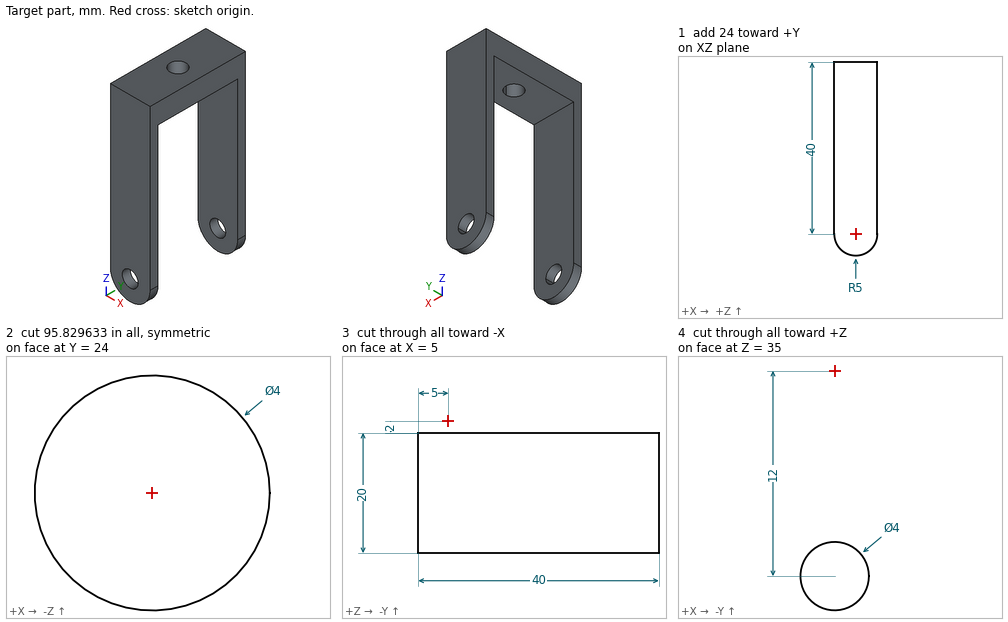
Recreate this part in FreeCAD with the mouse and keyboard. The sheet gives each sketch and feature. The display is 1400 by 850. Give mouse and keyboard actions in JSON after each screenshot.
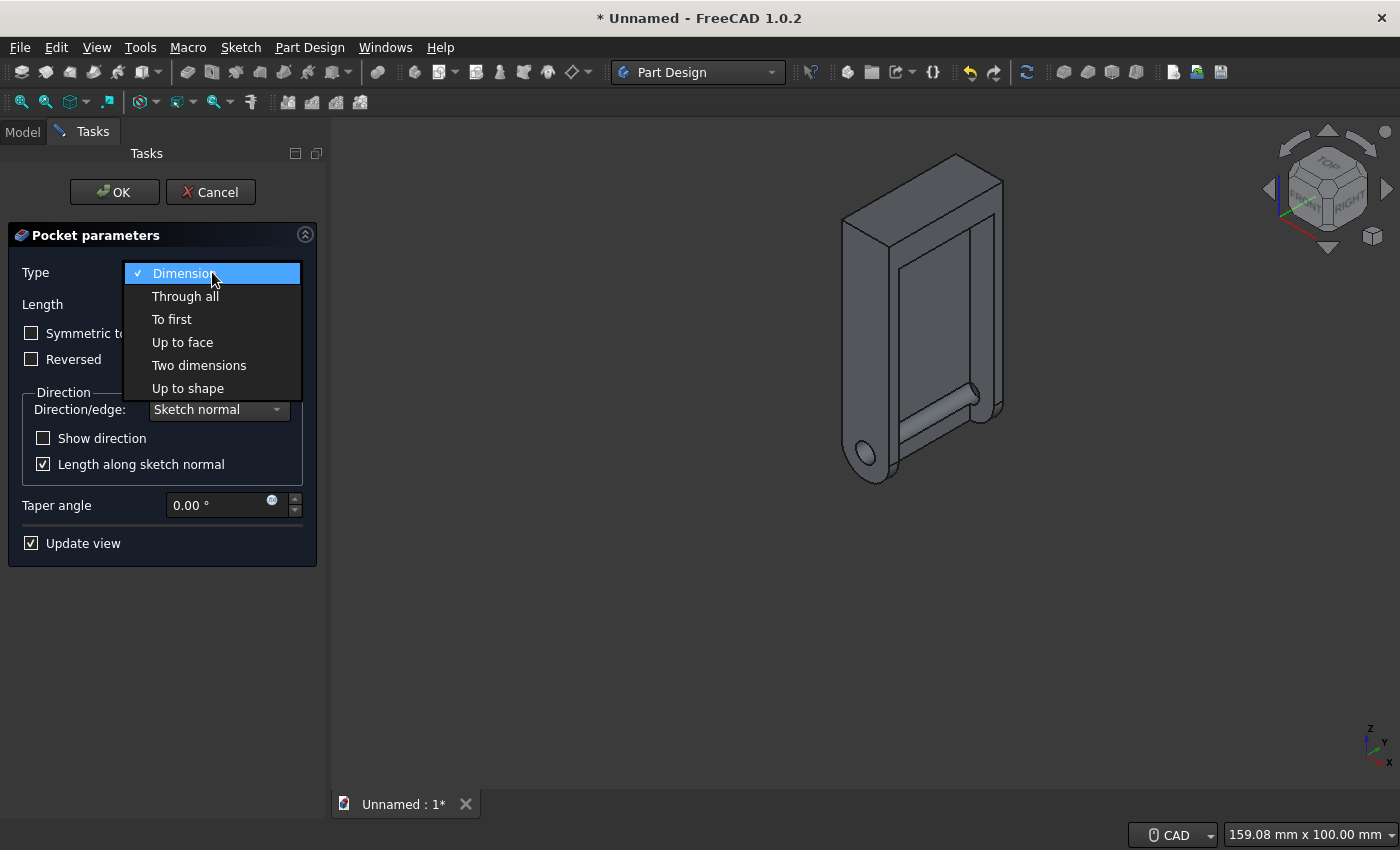
{"action": "left_click", "coordinate": [212, 296]}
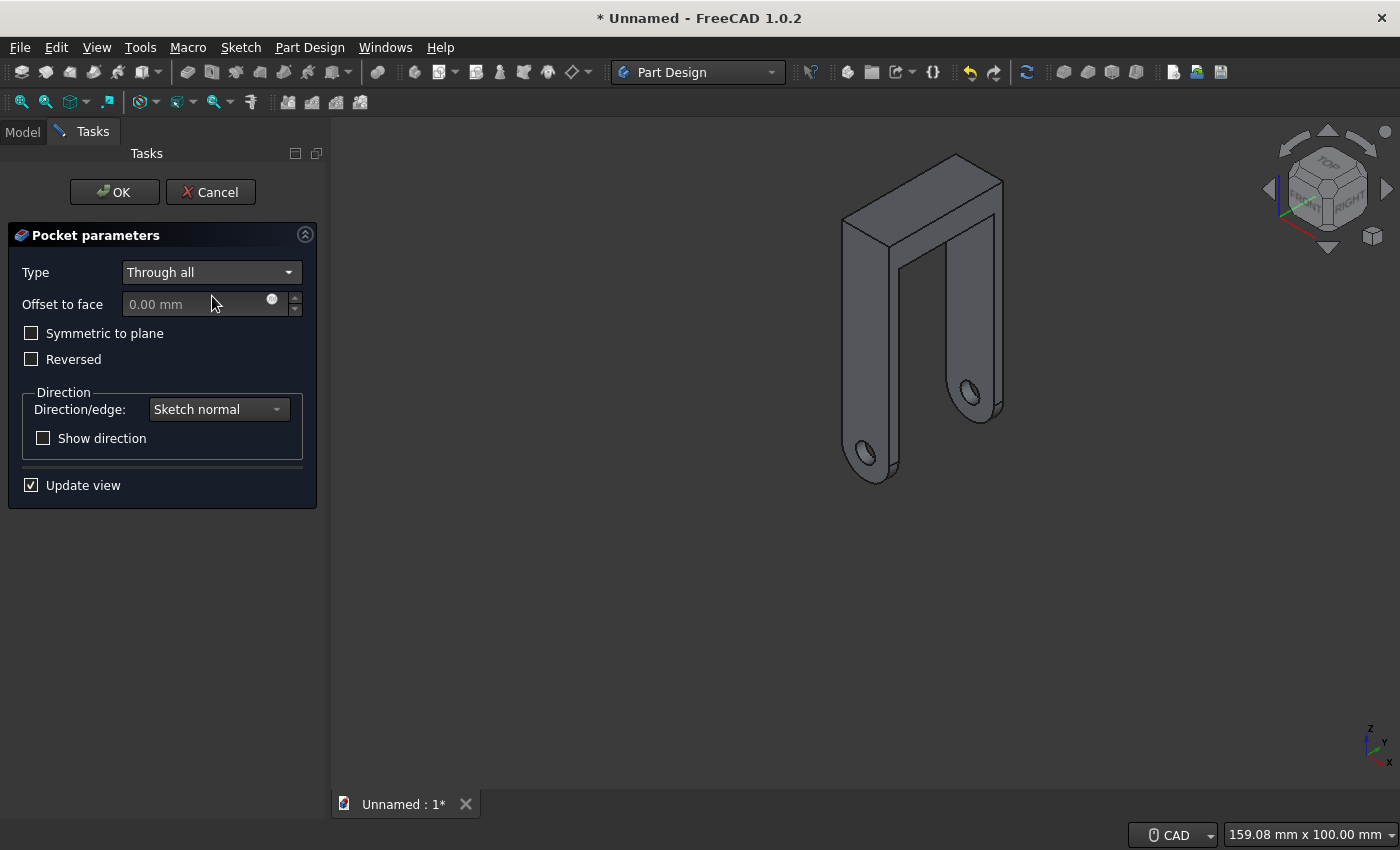
{"action": "left_click", "coordinate": [115, 192]}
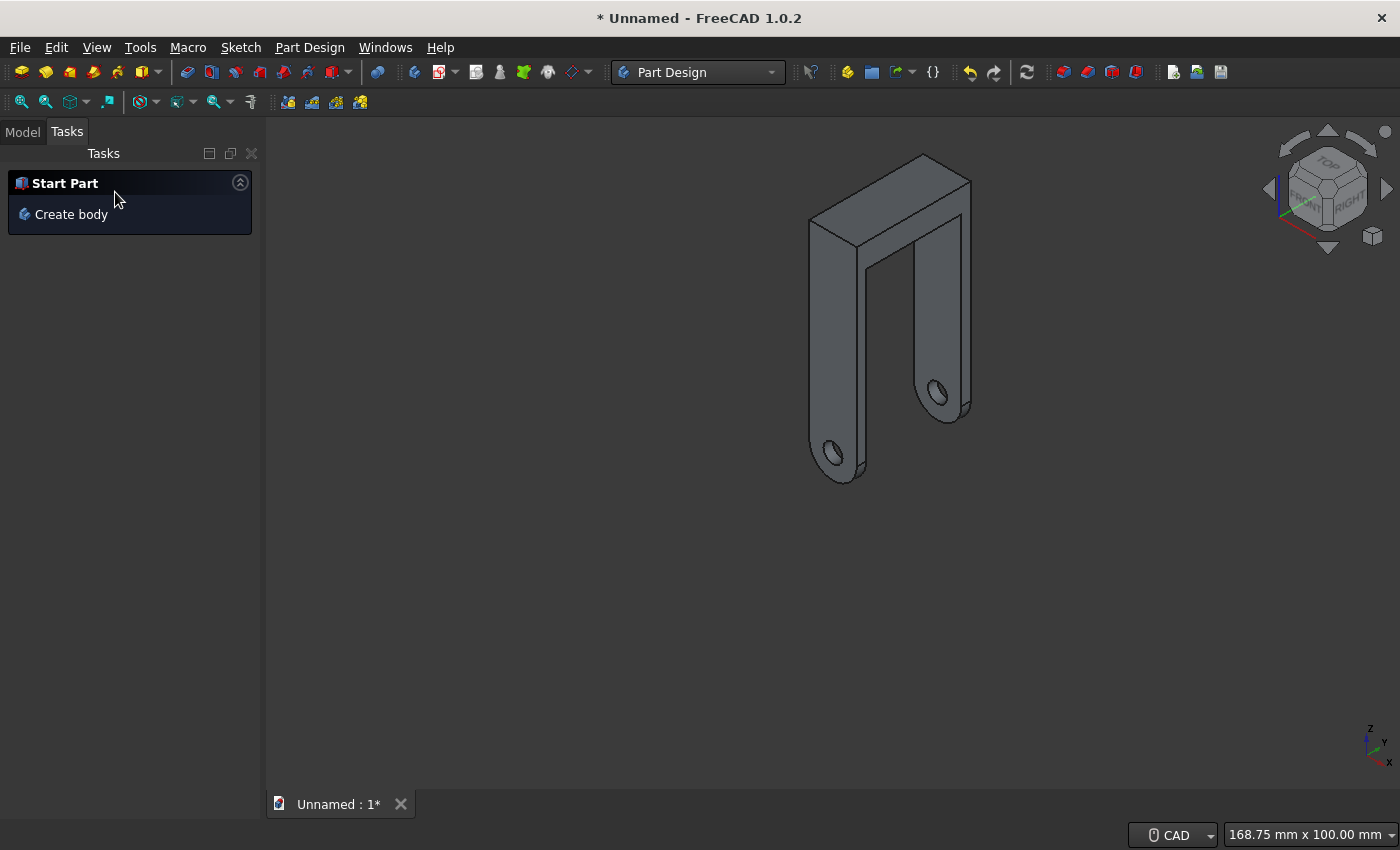
{"action": "key", "text": "5"}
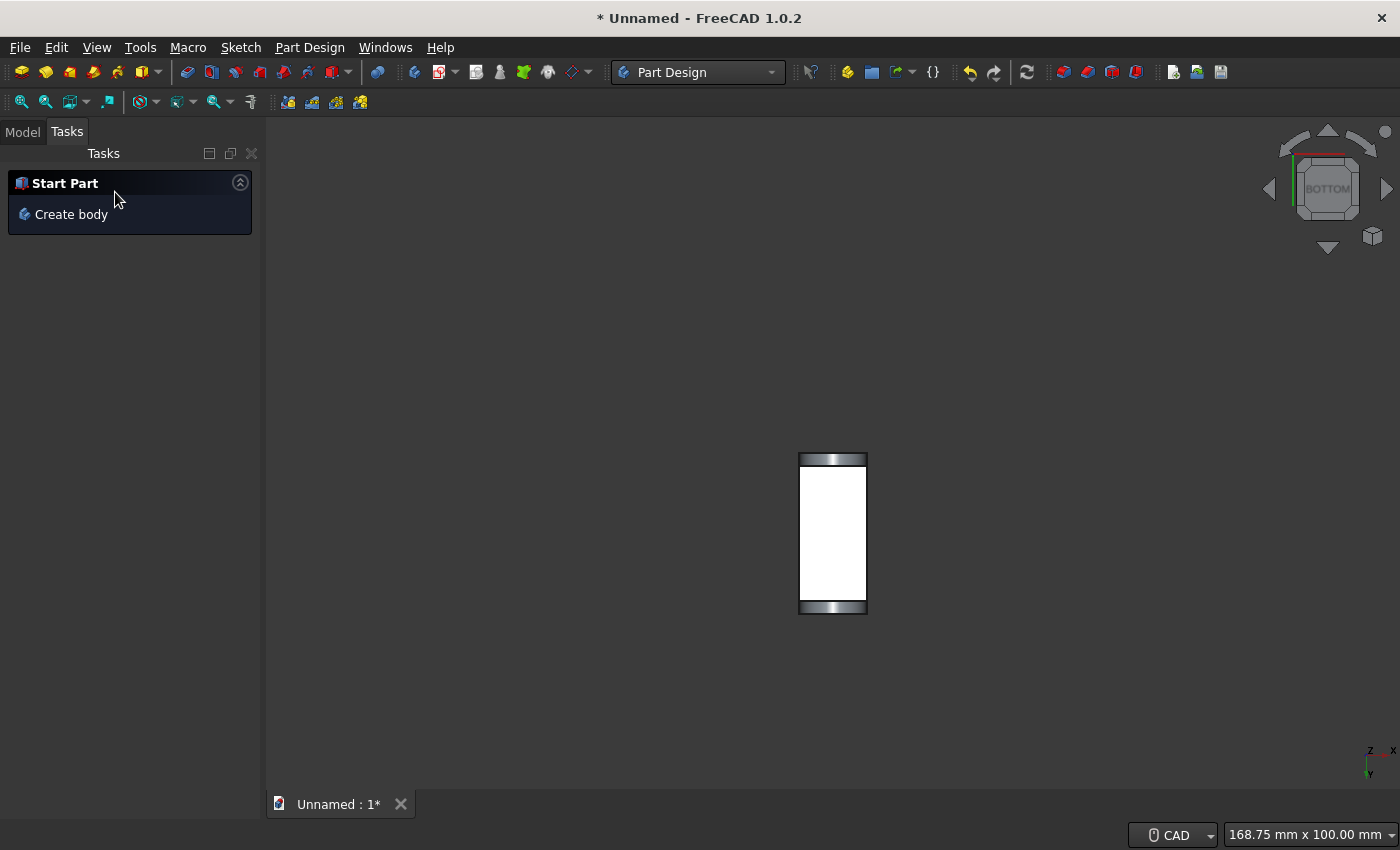
{"action": "key", "text": "v f"}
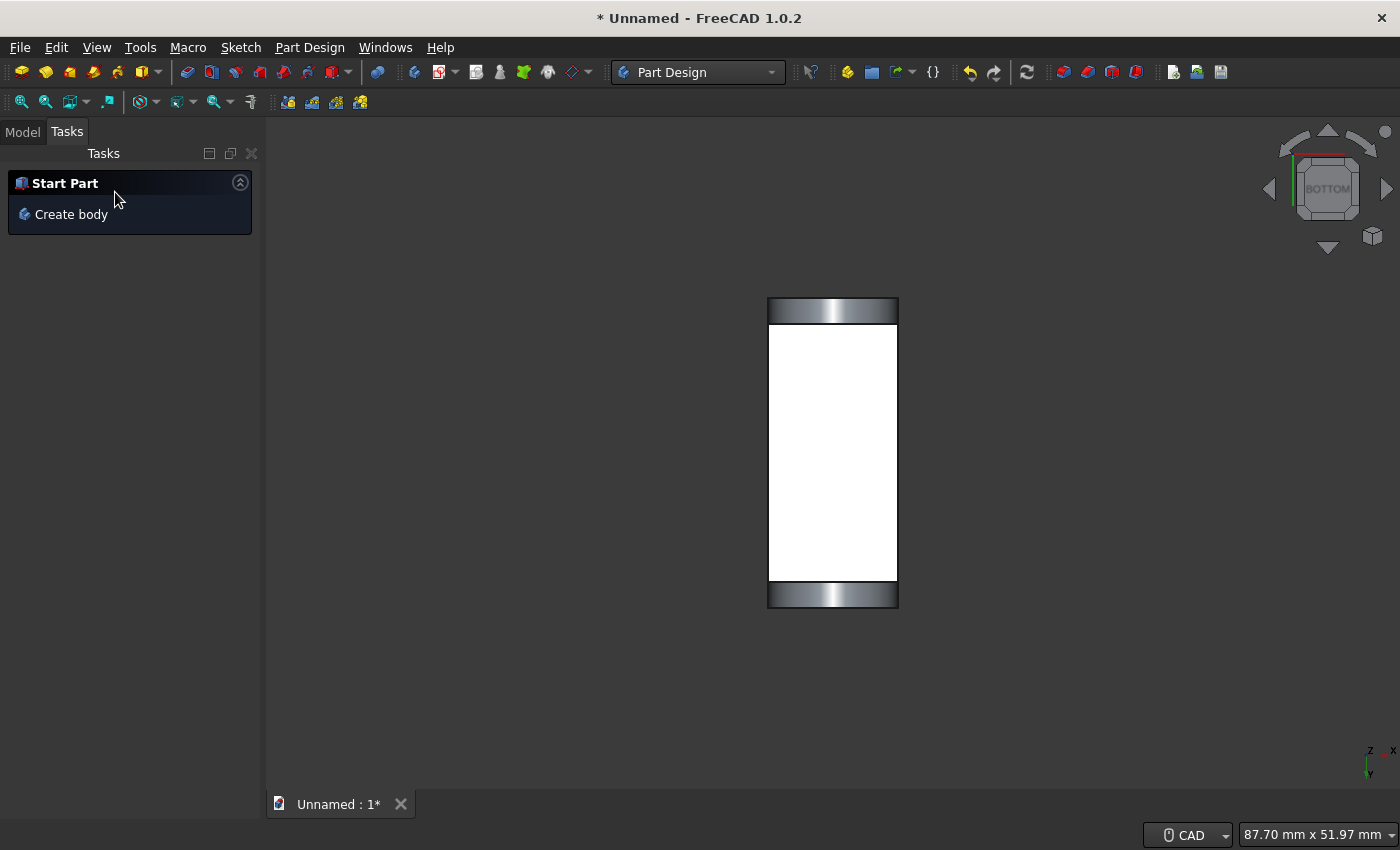
{"action": "left_click", "coordinate": [833, 489]}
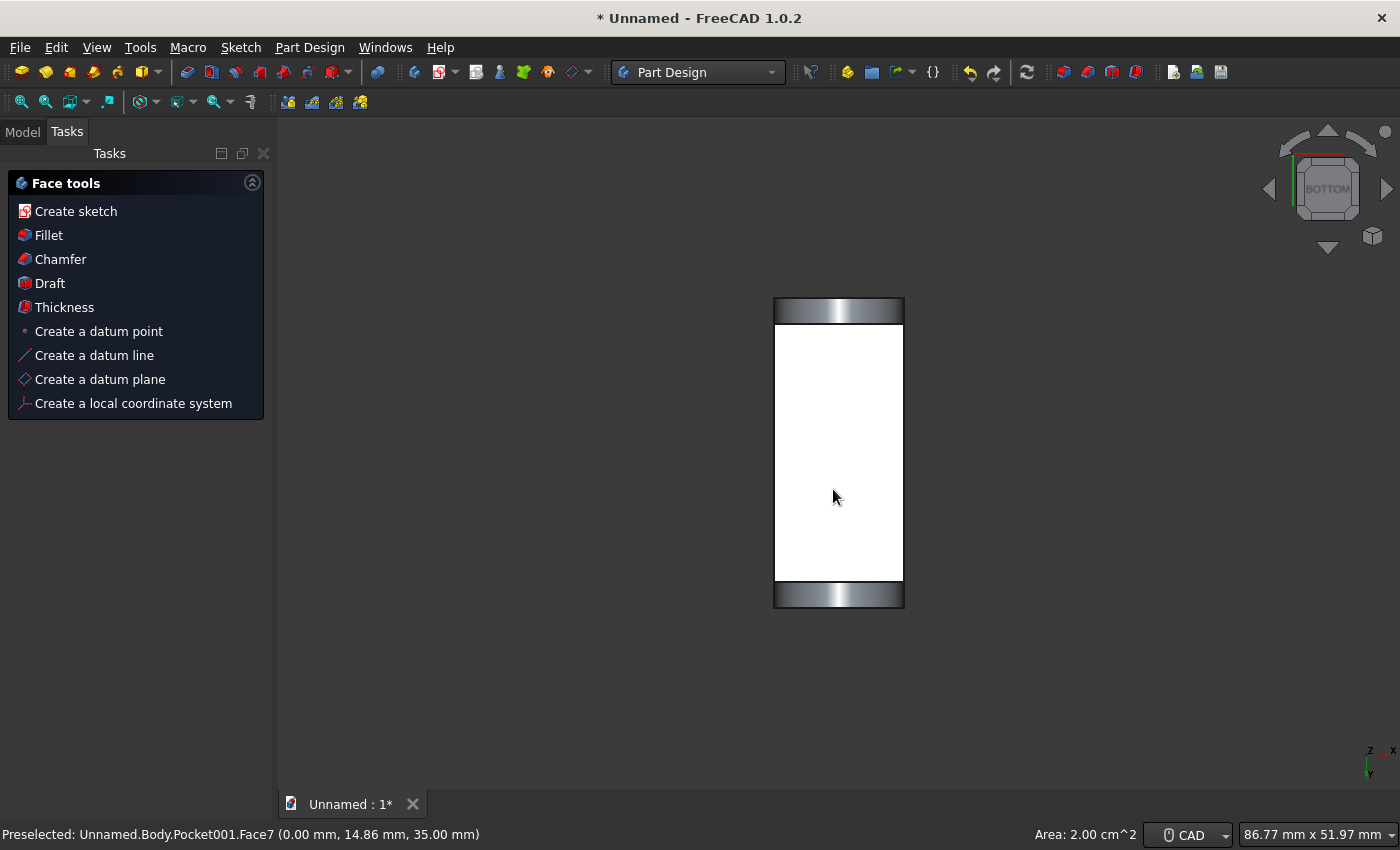
{"action": "left_click", "coordinate": [440, 72]}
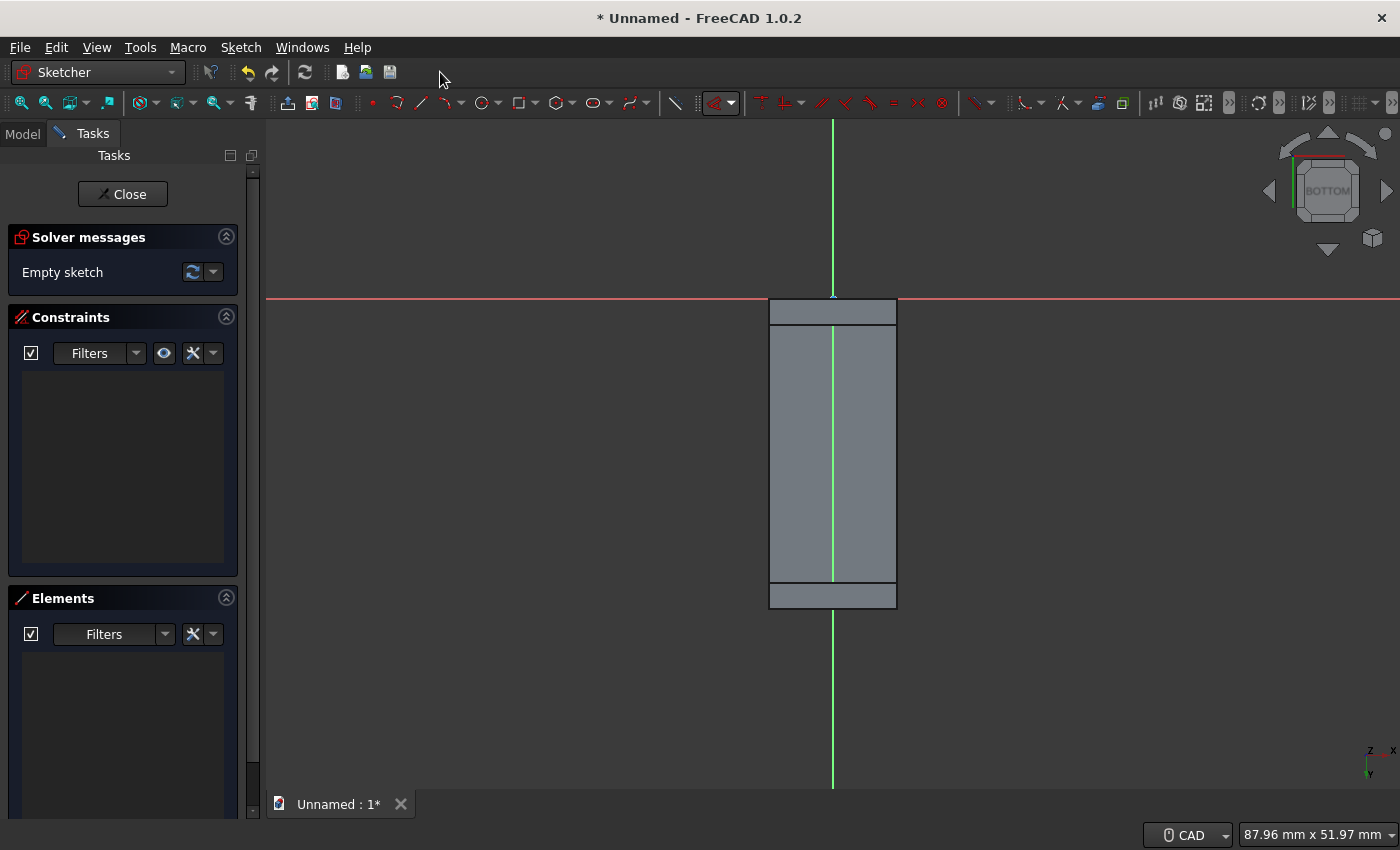
{"action": "scroll", "coordinate": [842, 454], "scroll_direction": "up", "scroll_amount": 11}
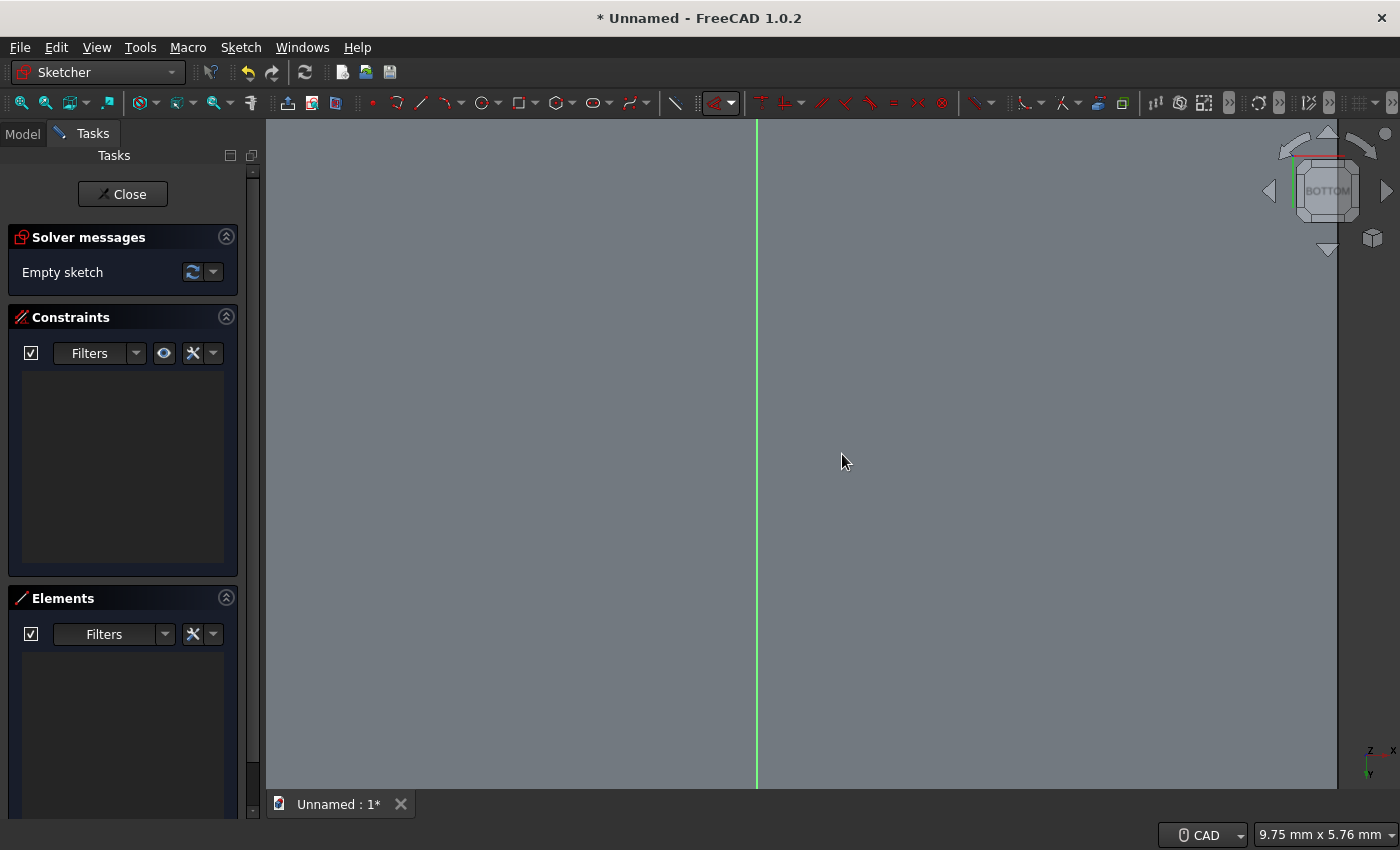
{"action": "key", "text": "g c"}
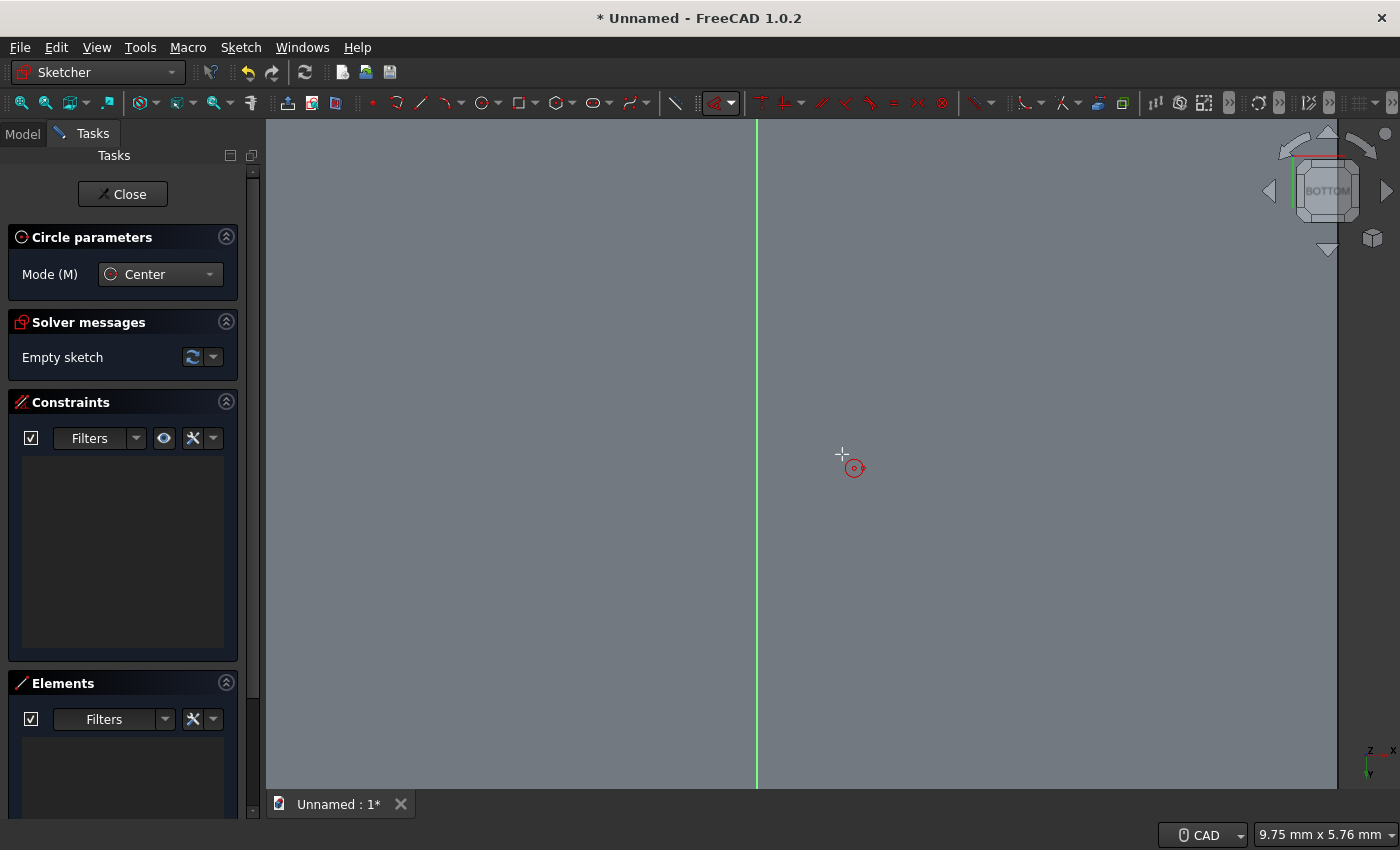
{"action": "left_click", "coordinate": [757, 450]}
{"action": "left_click", "coordinate": [921, 285]}
{"action": "key", "text": "Escape"}